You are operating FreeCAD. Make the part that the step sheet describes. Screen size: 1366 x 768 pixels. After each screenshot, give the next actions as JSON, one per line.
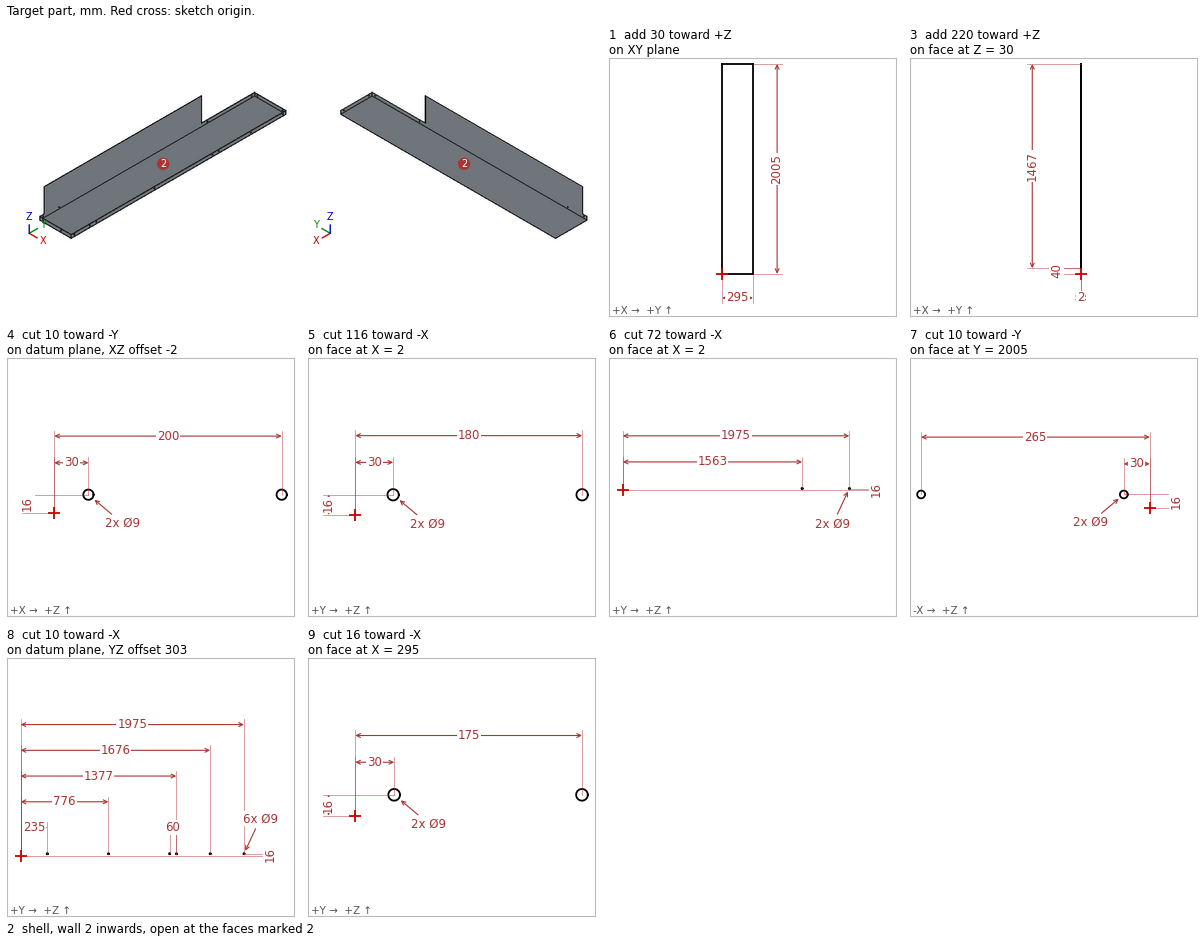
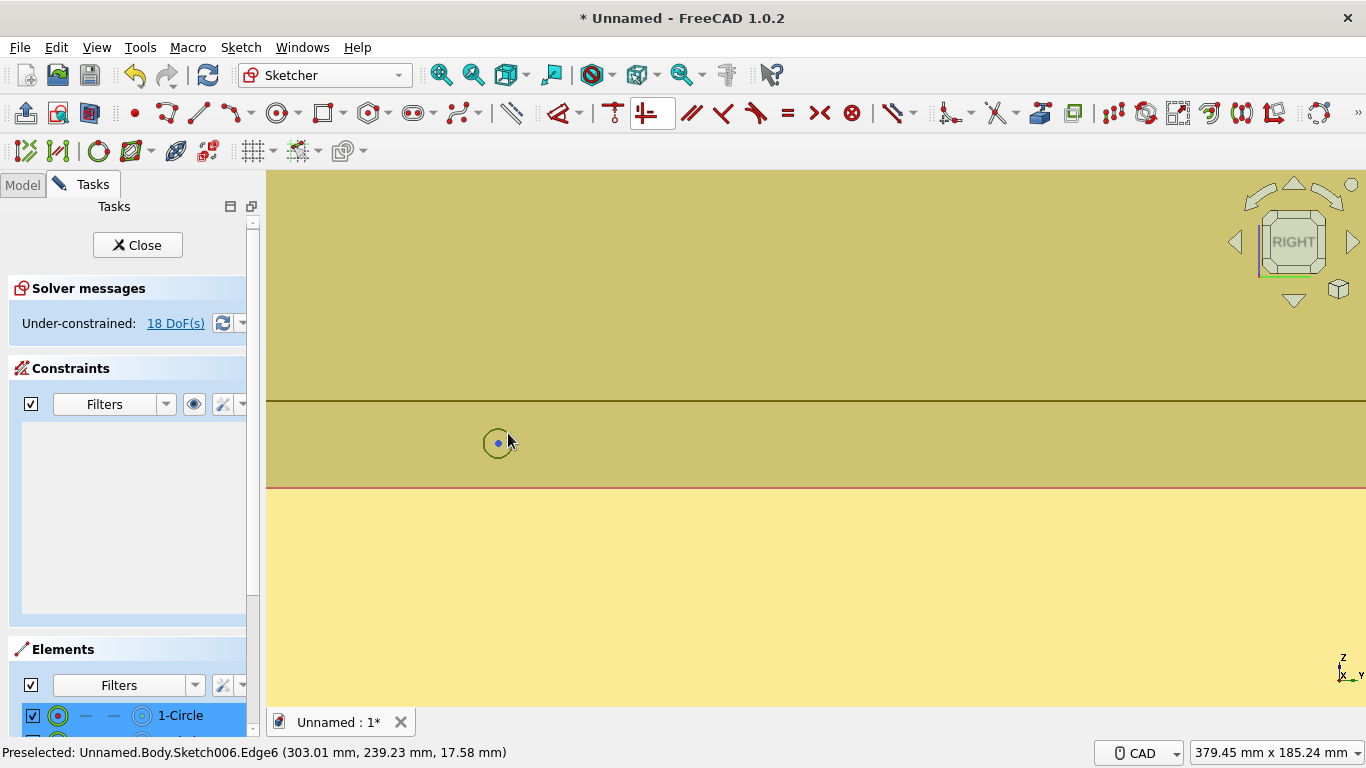
{"action": "key", "text": "e"}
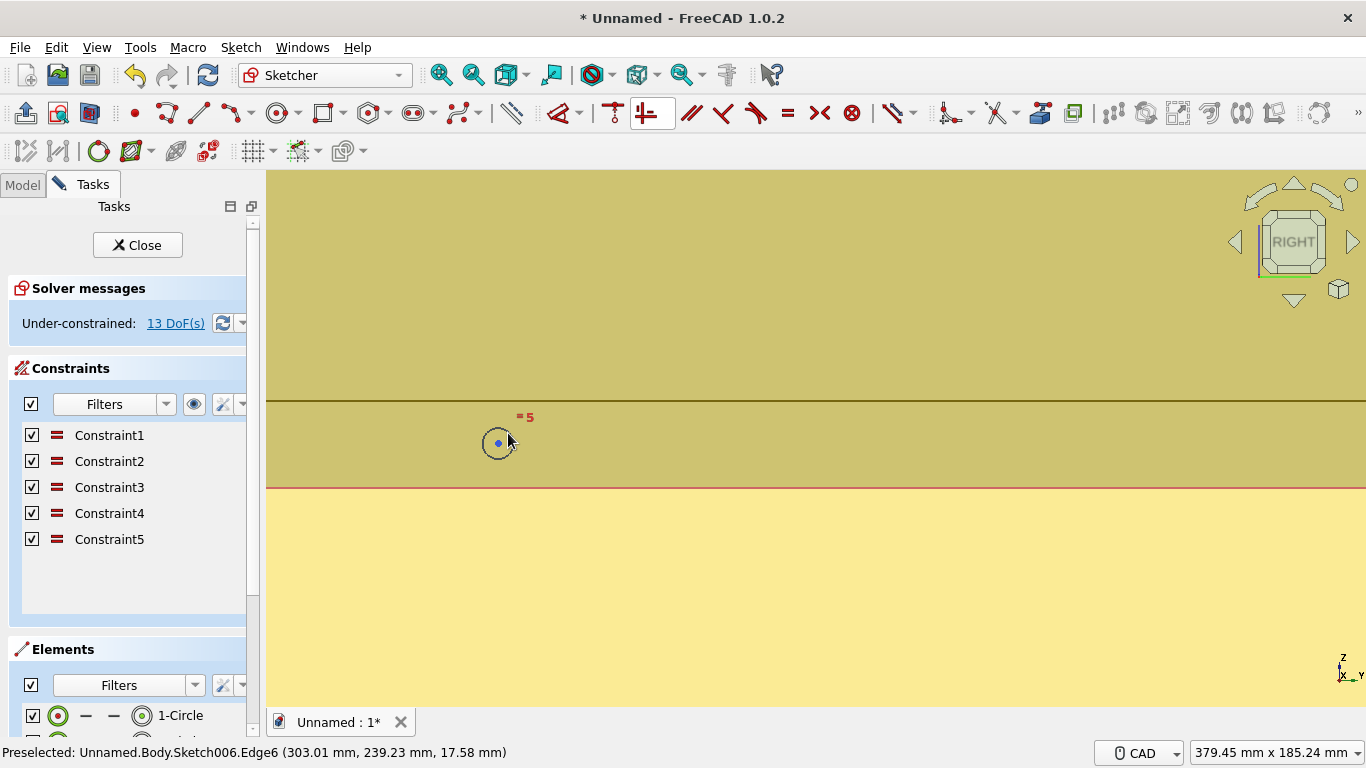
{"action": "scroll", "coordinate": [506, 436], "scroll_direction": "down", "scroll_amount": 11}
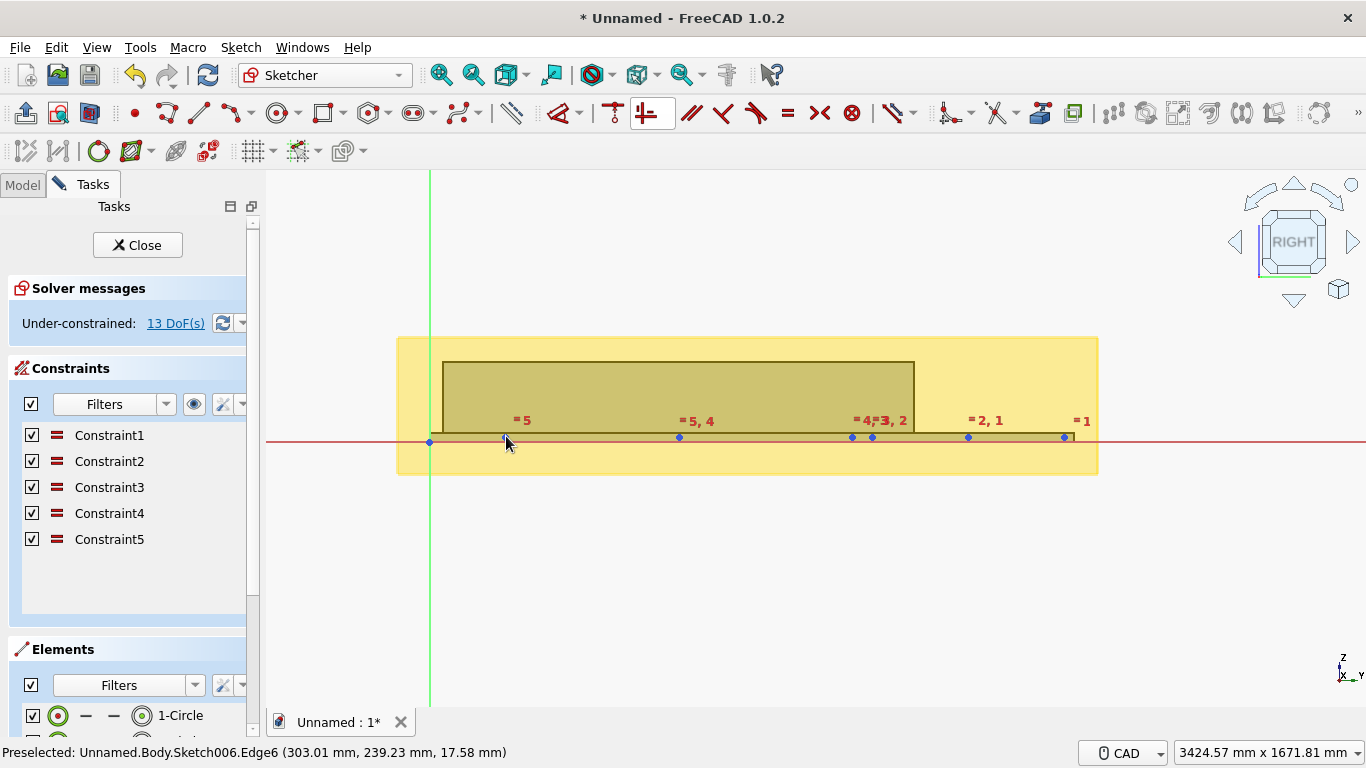
{"action": "left_click", "coordinate": [1064, 437]}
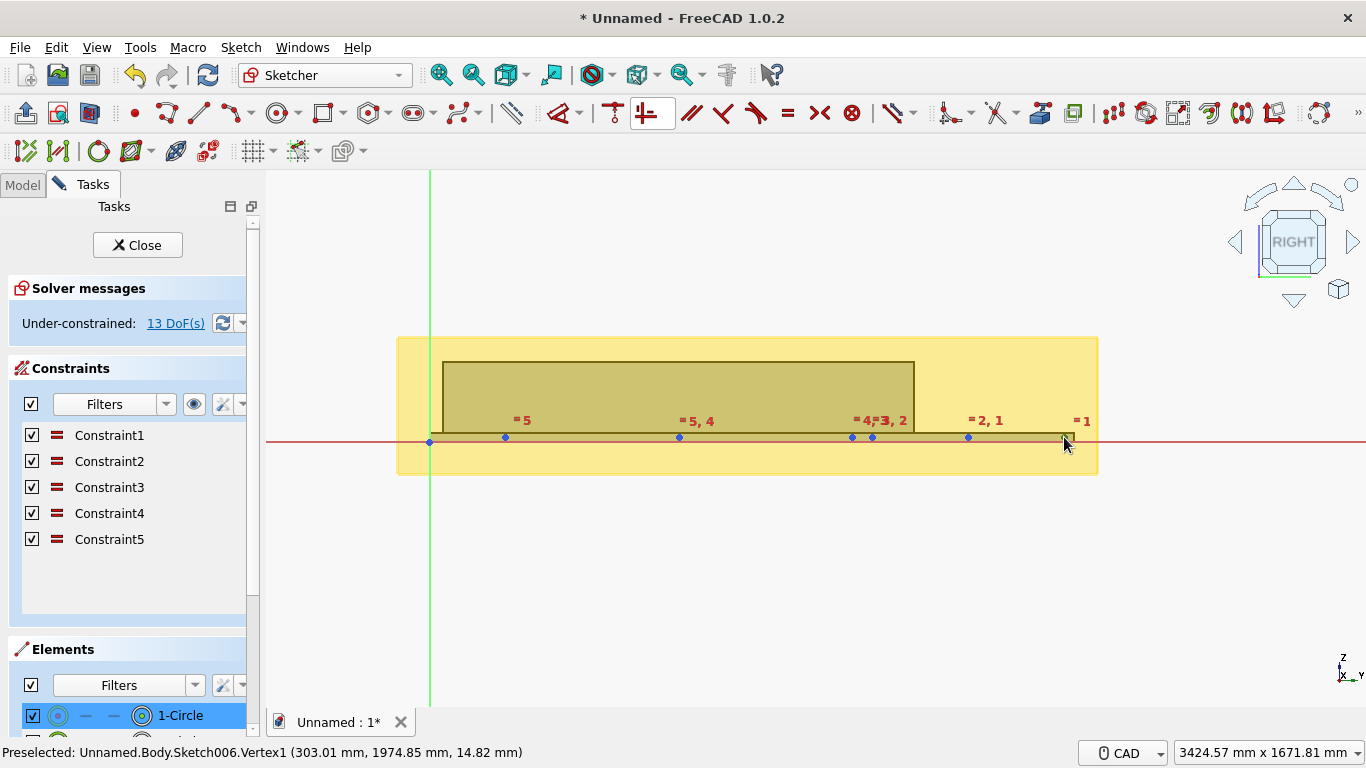
{"action": "left_click", "coordinate": [968, 437]}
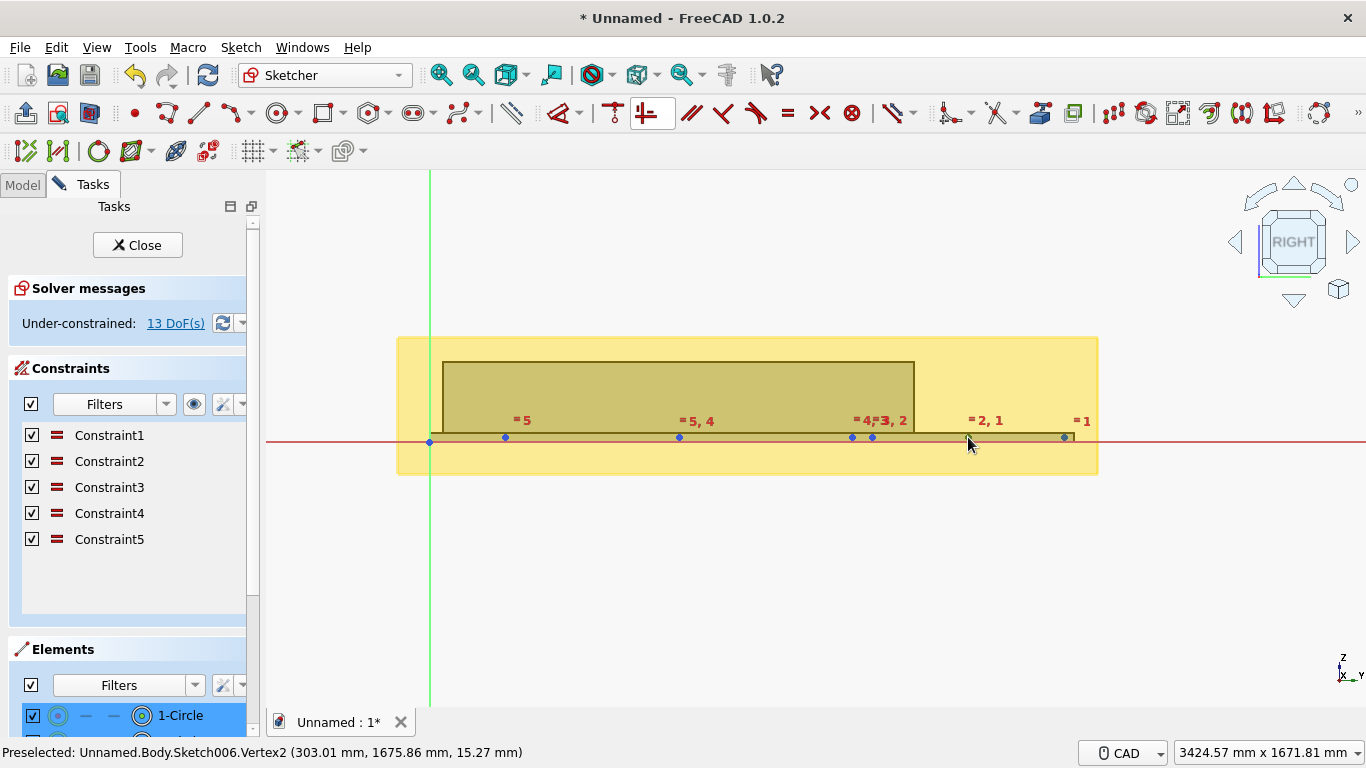
{"action": "key", "text": "h"}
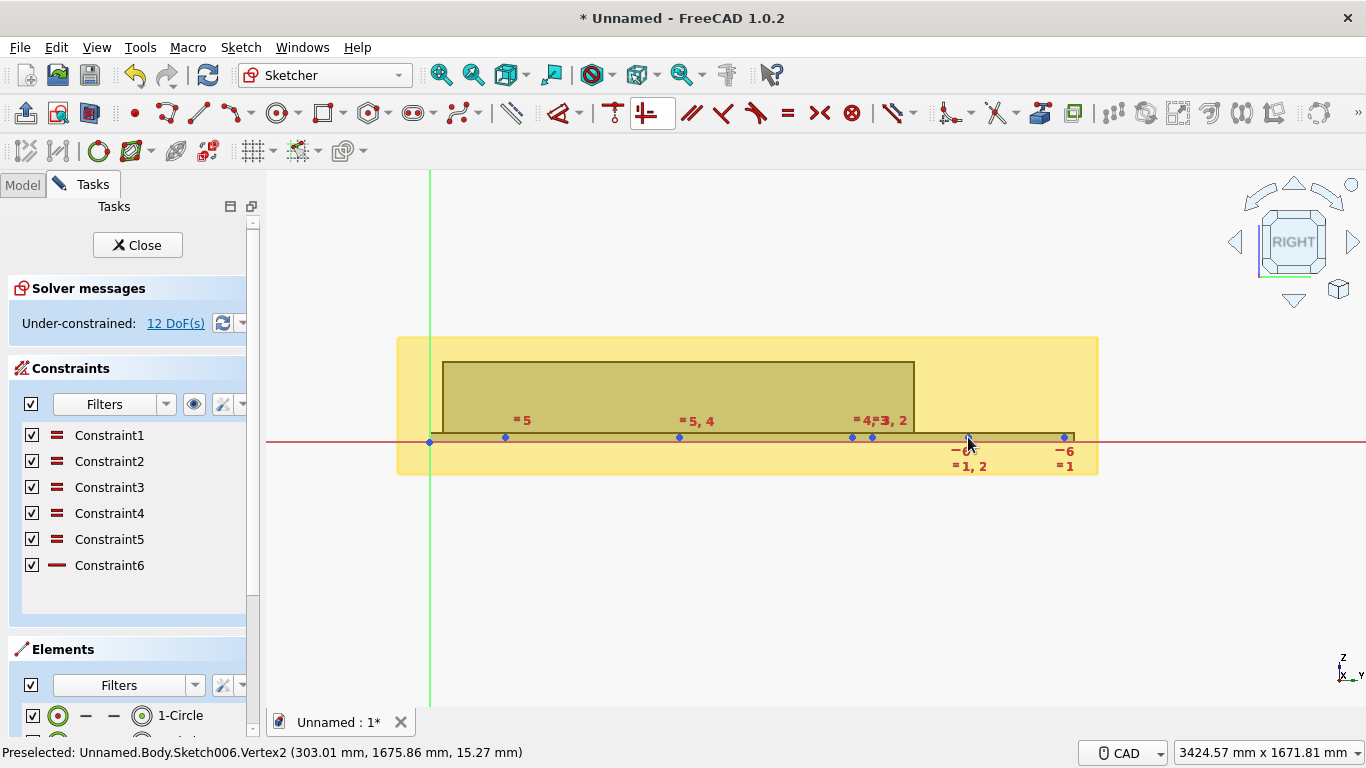
{"action": "left_click", "coordinate": [968, 437]}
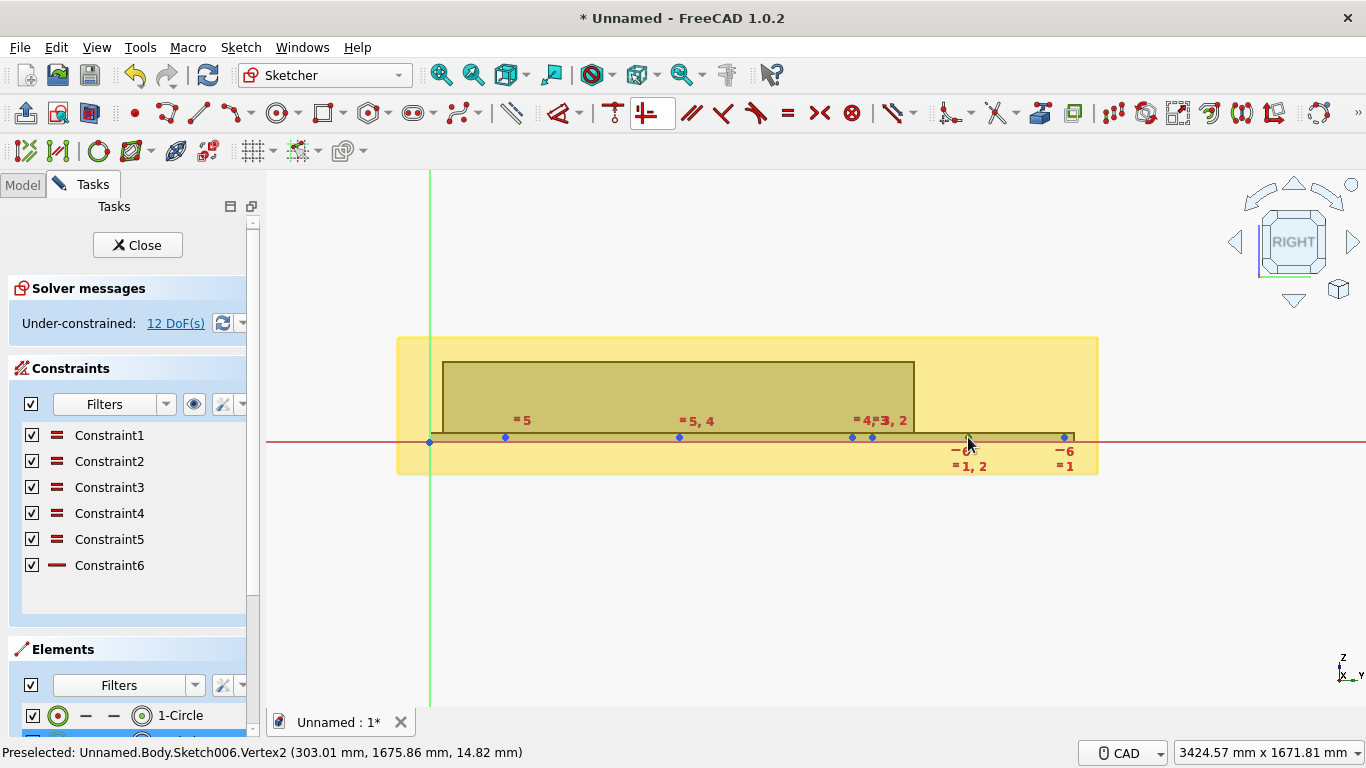
{"action": "left_click", "coordinate": [872, 437]}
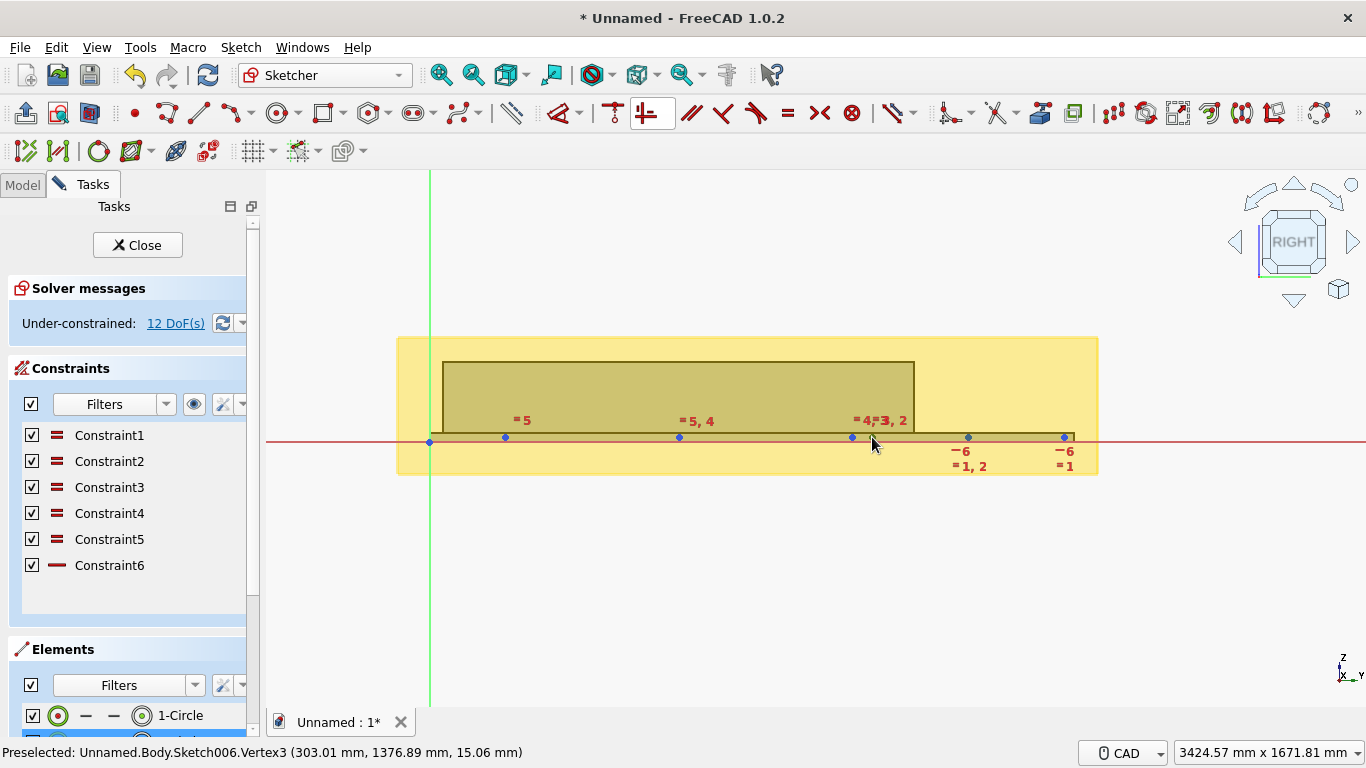
{"action": "left_click", "coordinate": [670, 114]}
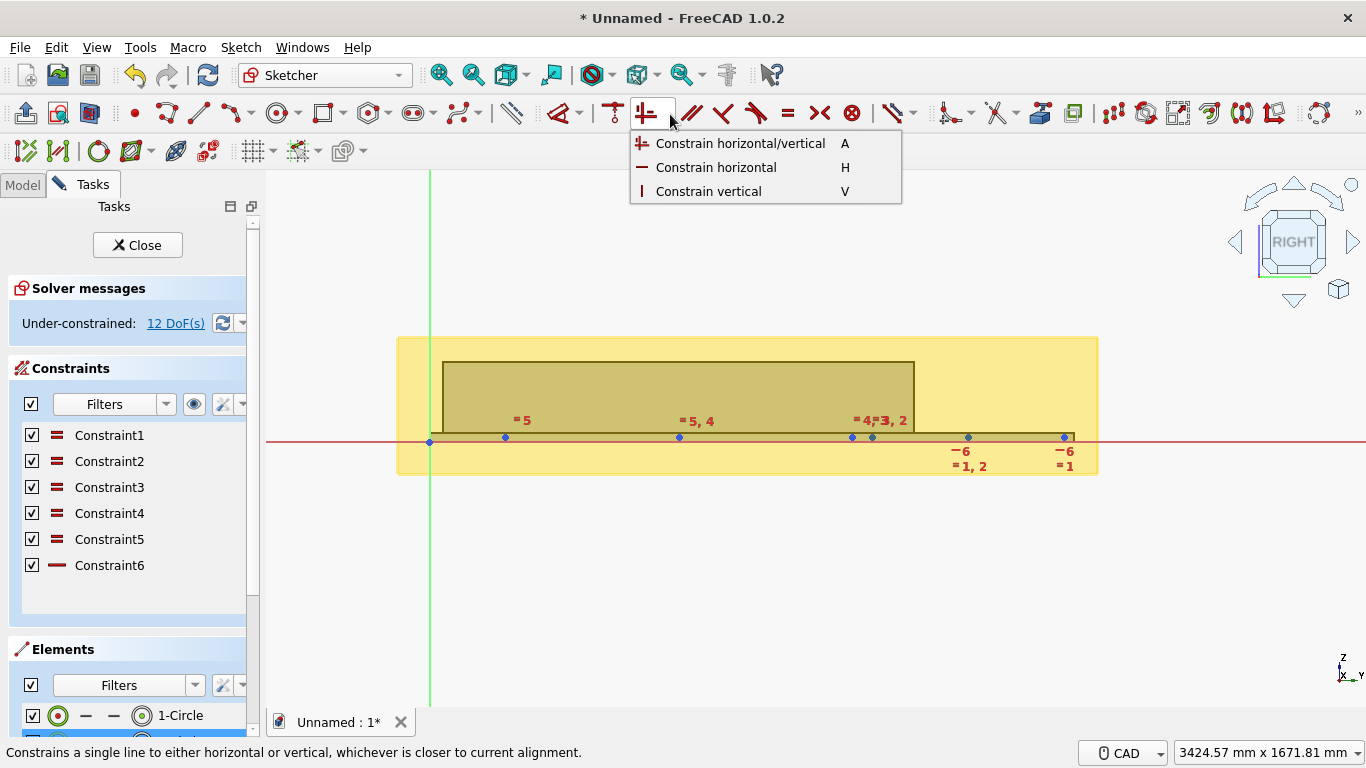
{"action": "left_click", "coordinate": [766, 167]}